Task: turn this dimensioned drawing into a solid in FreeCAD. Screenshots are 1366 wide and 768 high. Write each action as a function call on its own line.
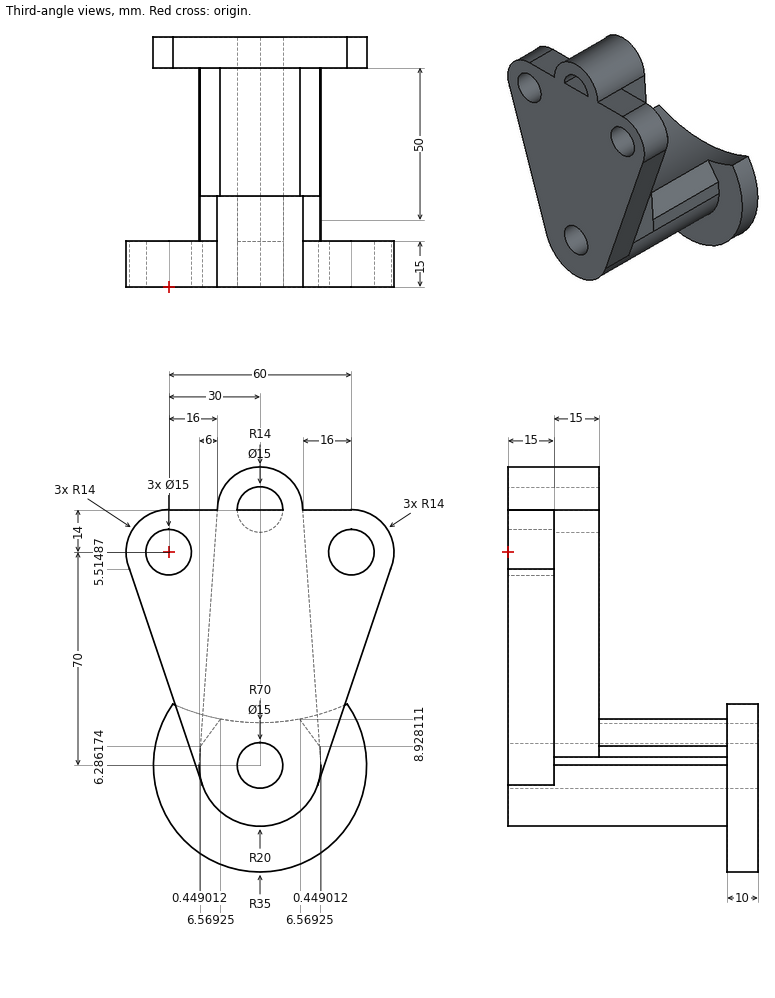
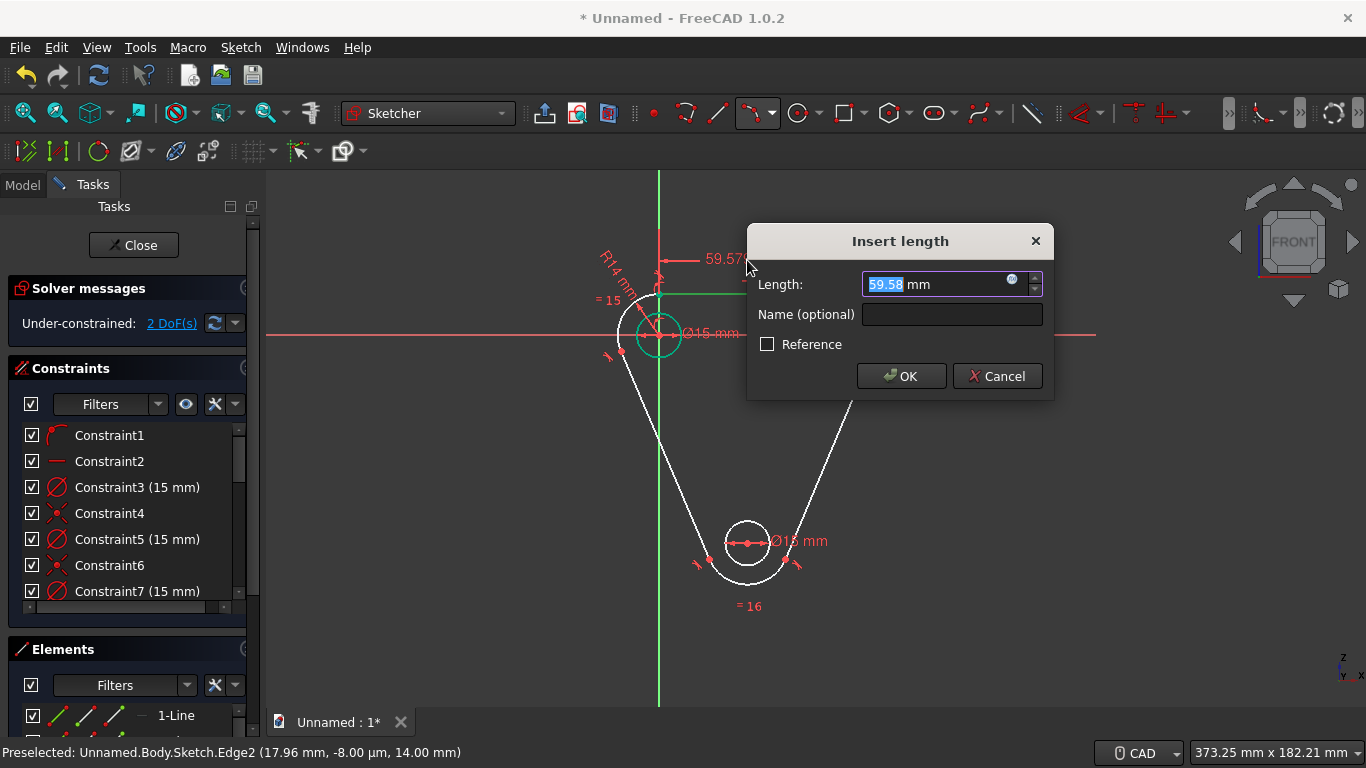
text(60)
key(Return)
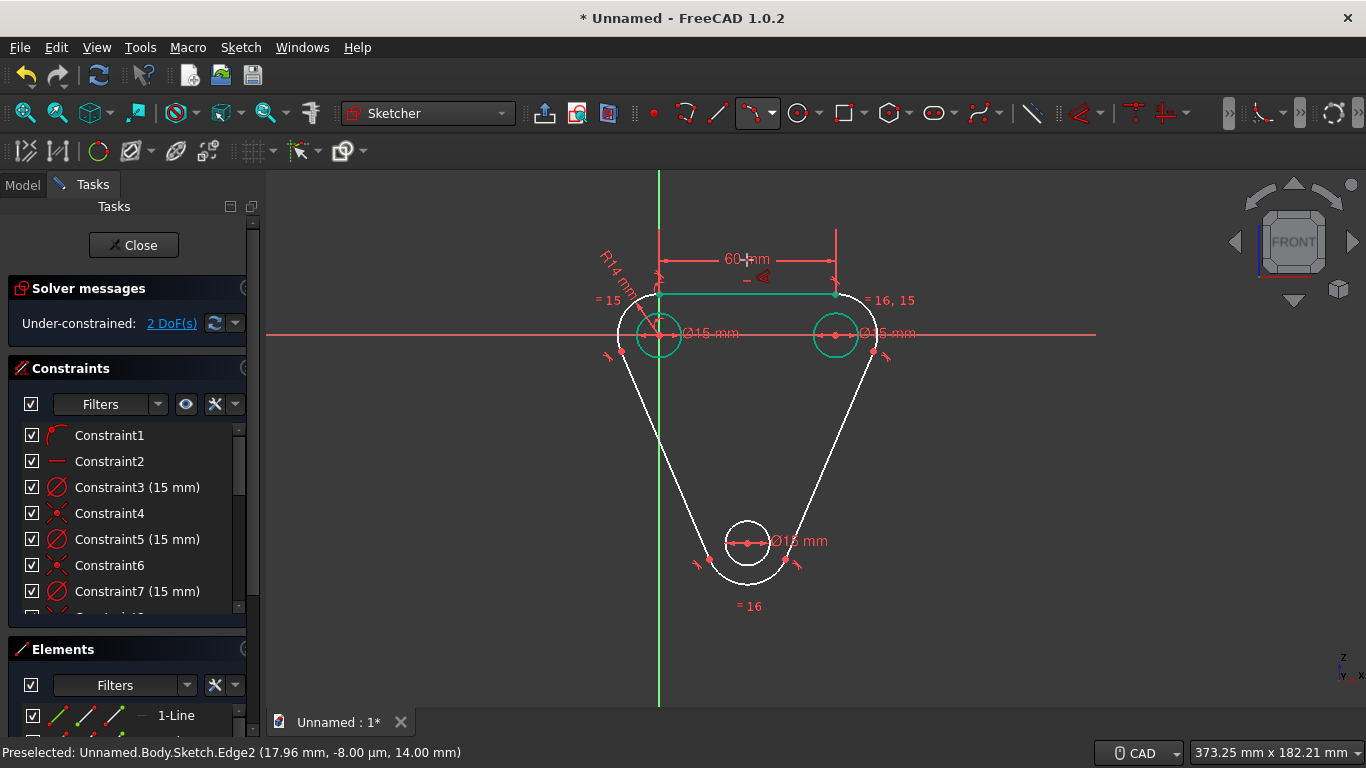
click(748, 543)
click(703, 577)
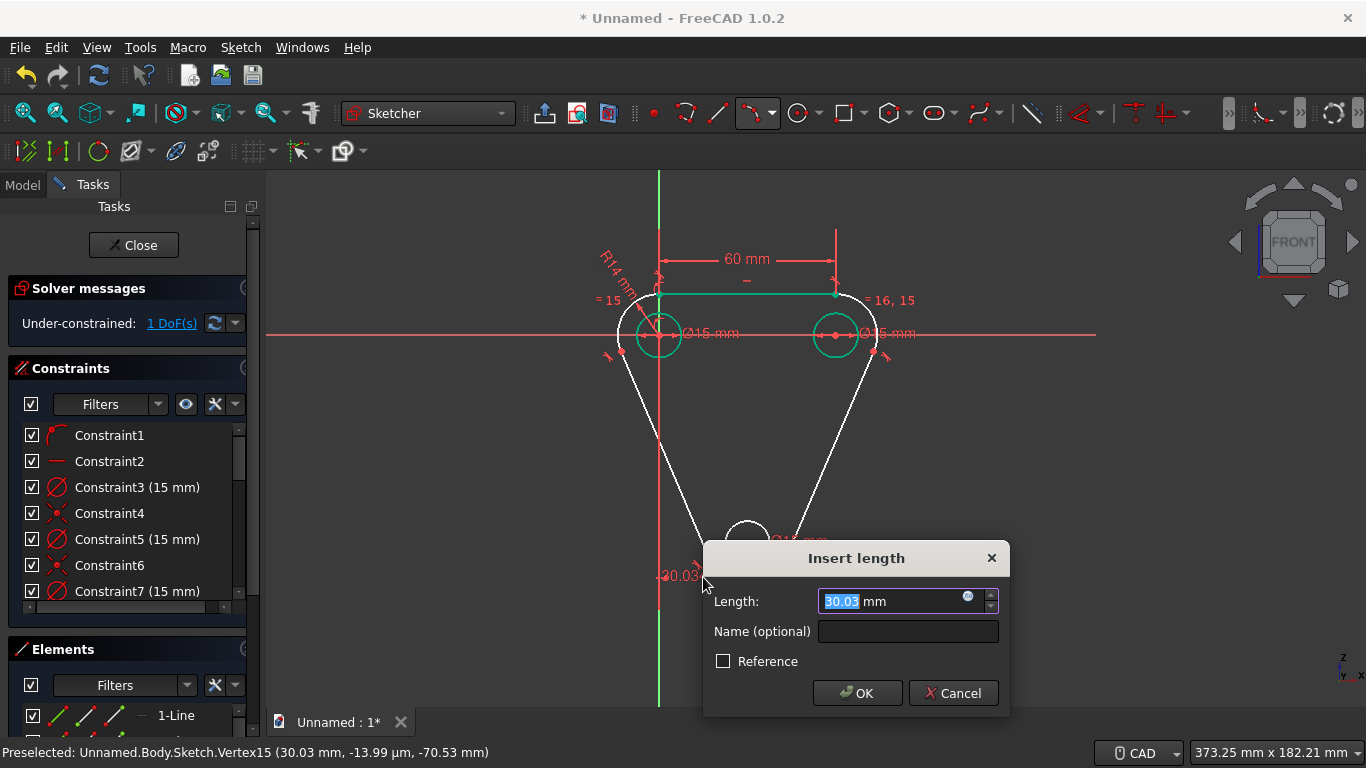
text(30)
key(Return)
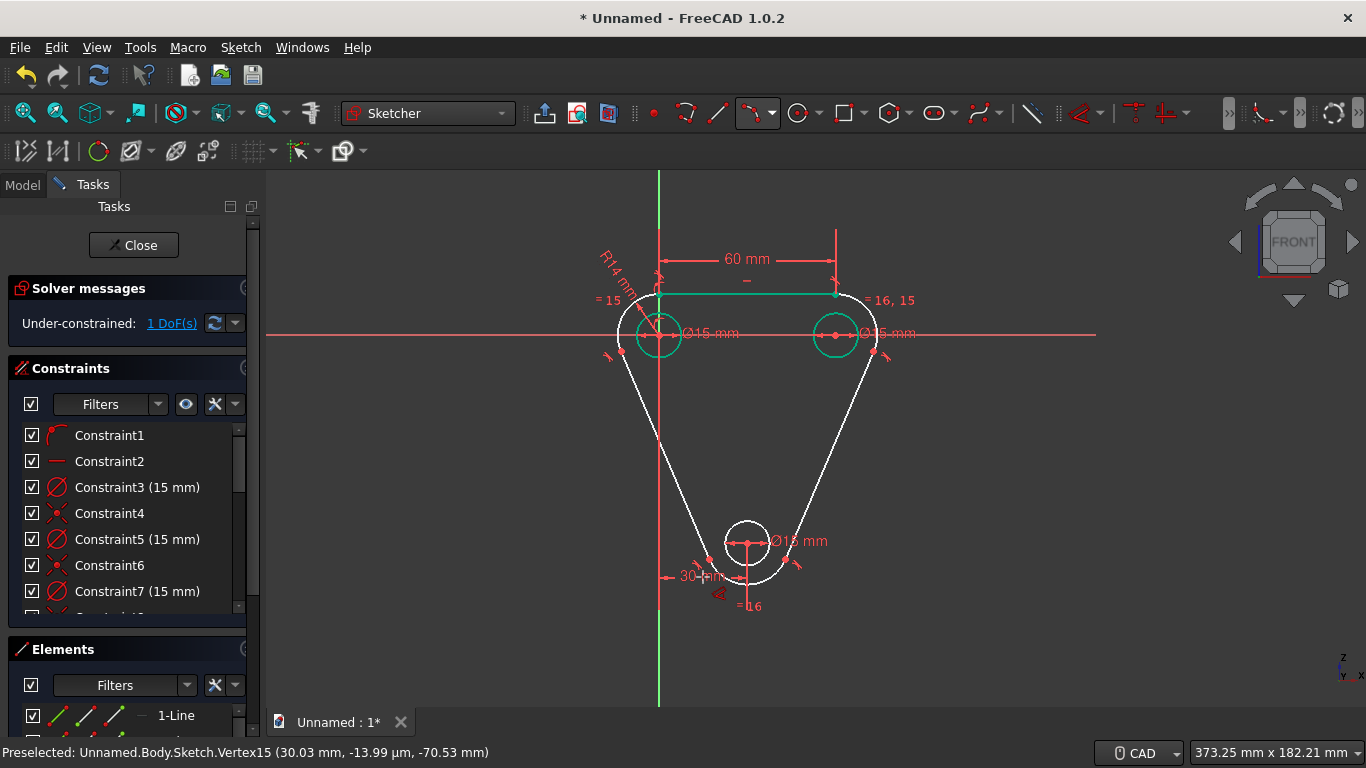
click(747, 543)
click(625, 439)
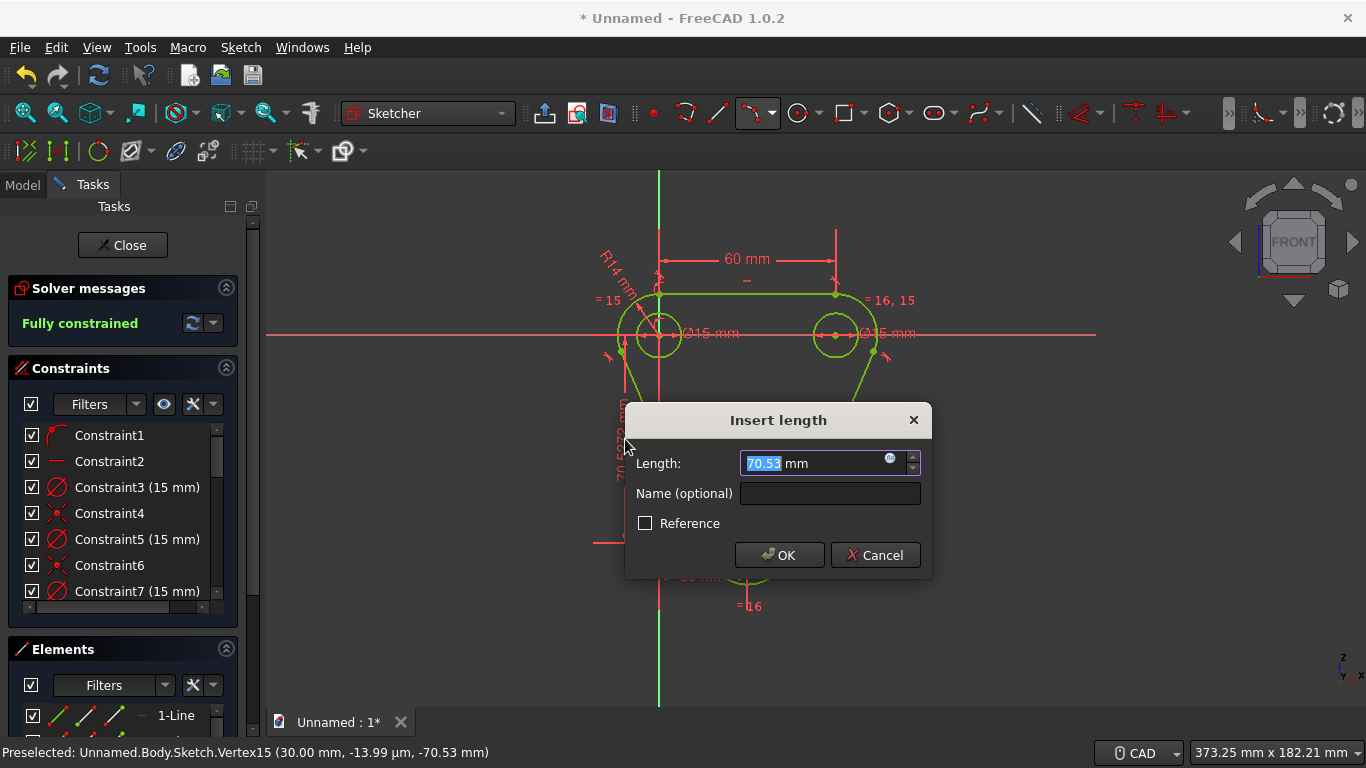
text(70)
key(Return)
key(Escape)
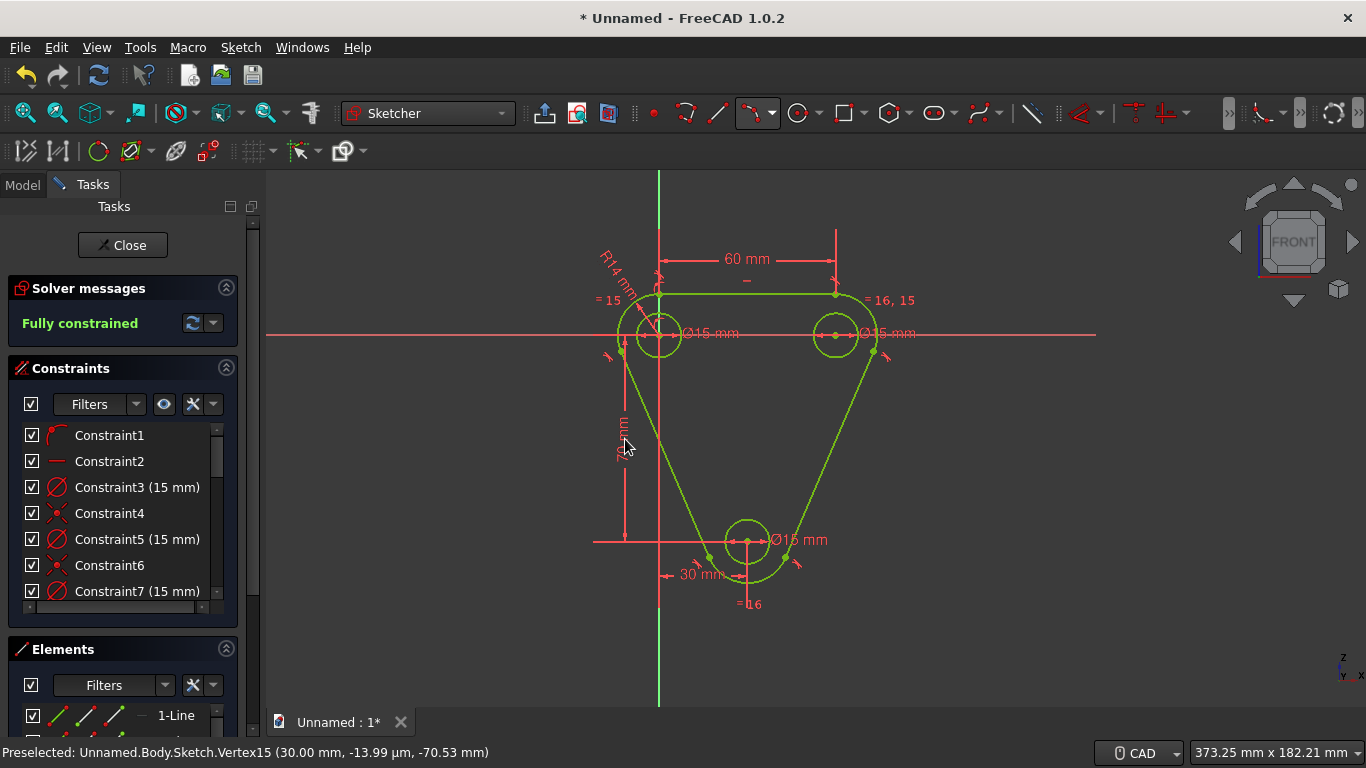
click(123, 245)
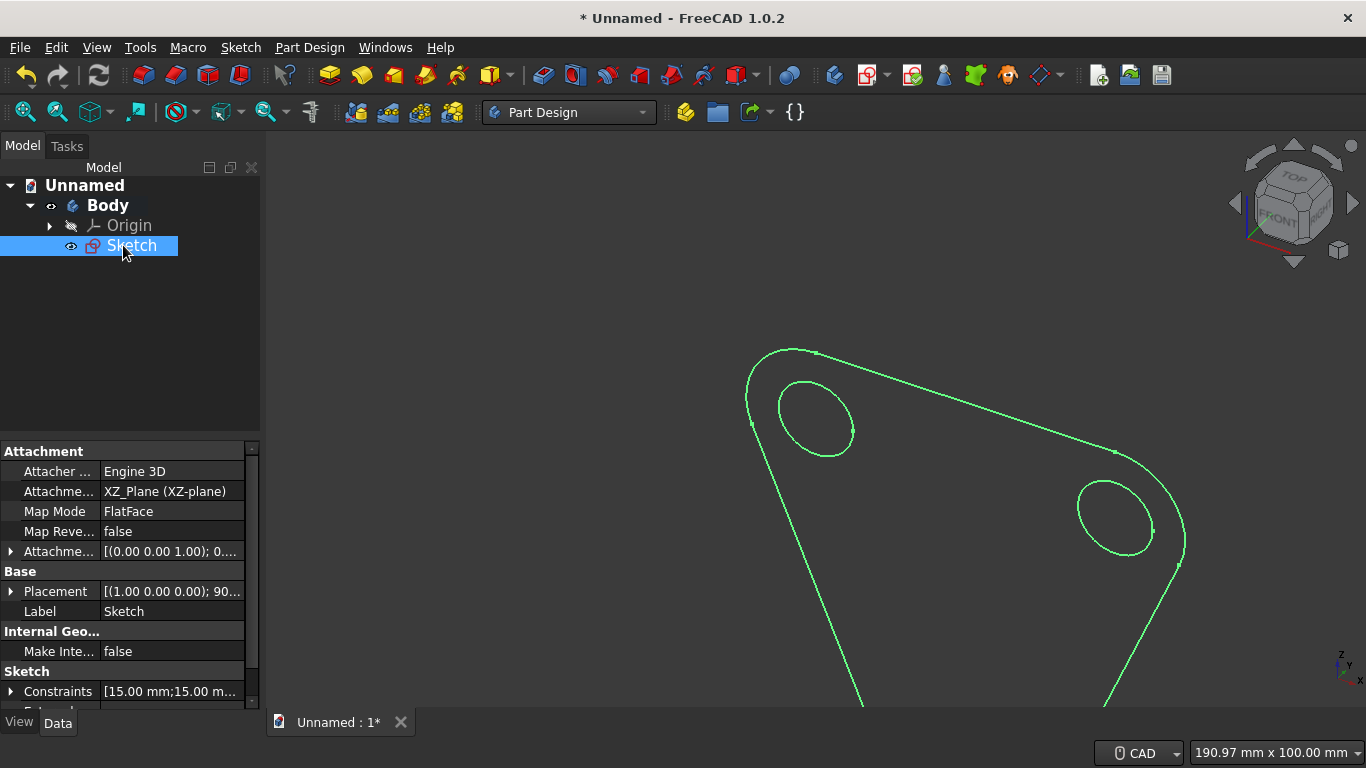
click(330, 76)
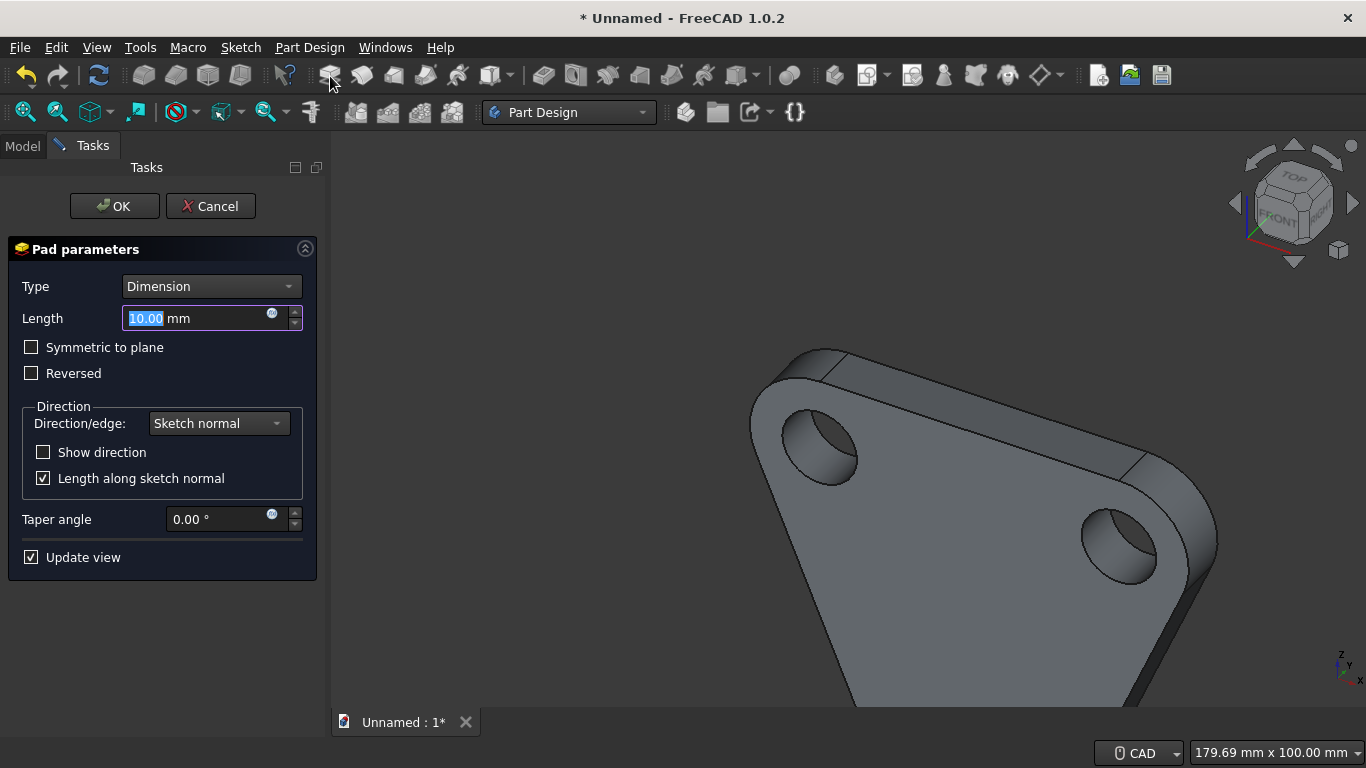
text(15)
key(Tab)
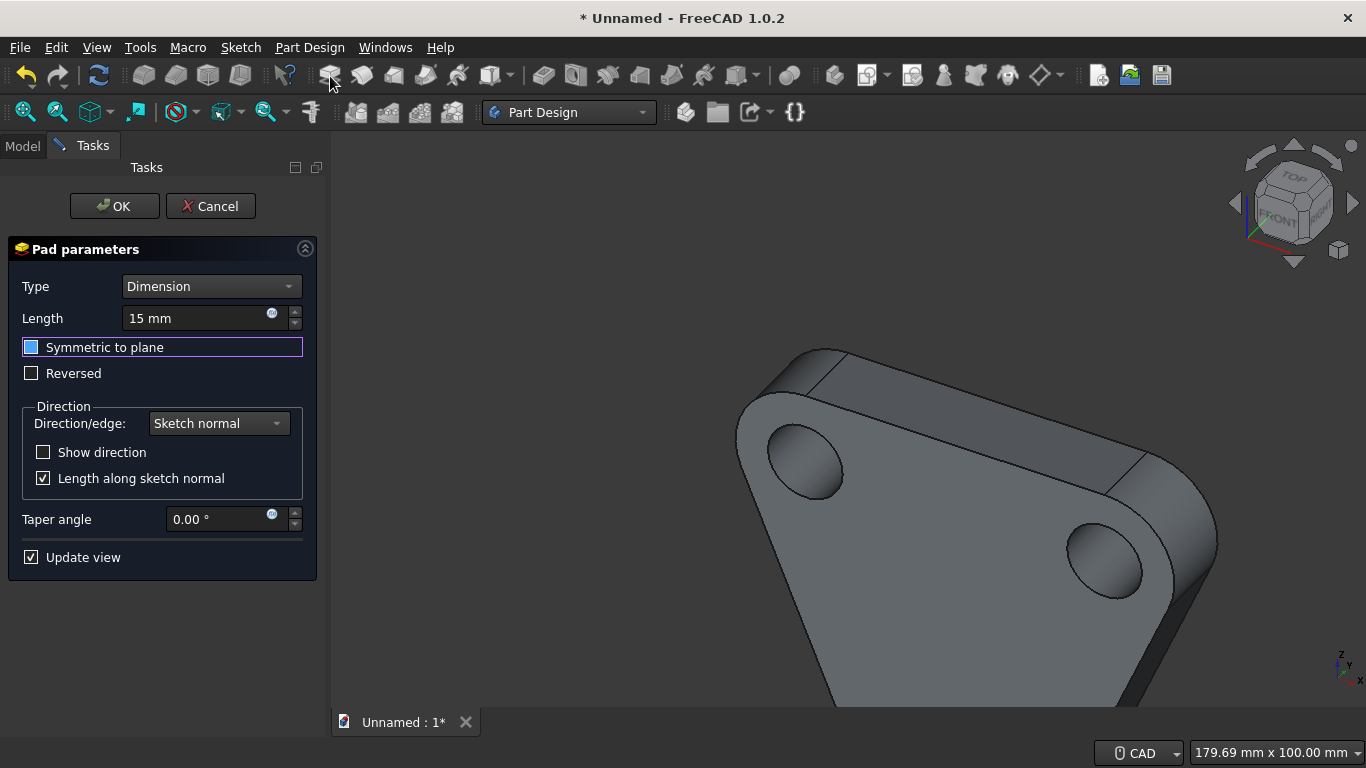
click(30, 373)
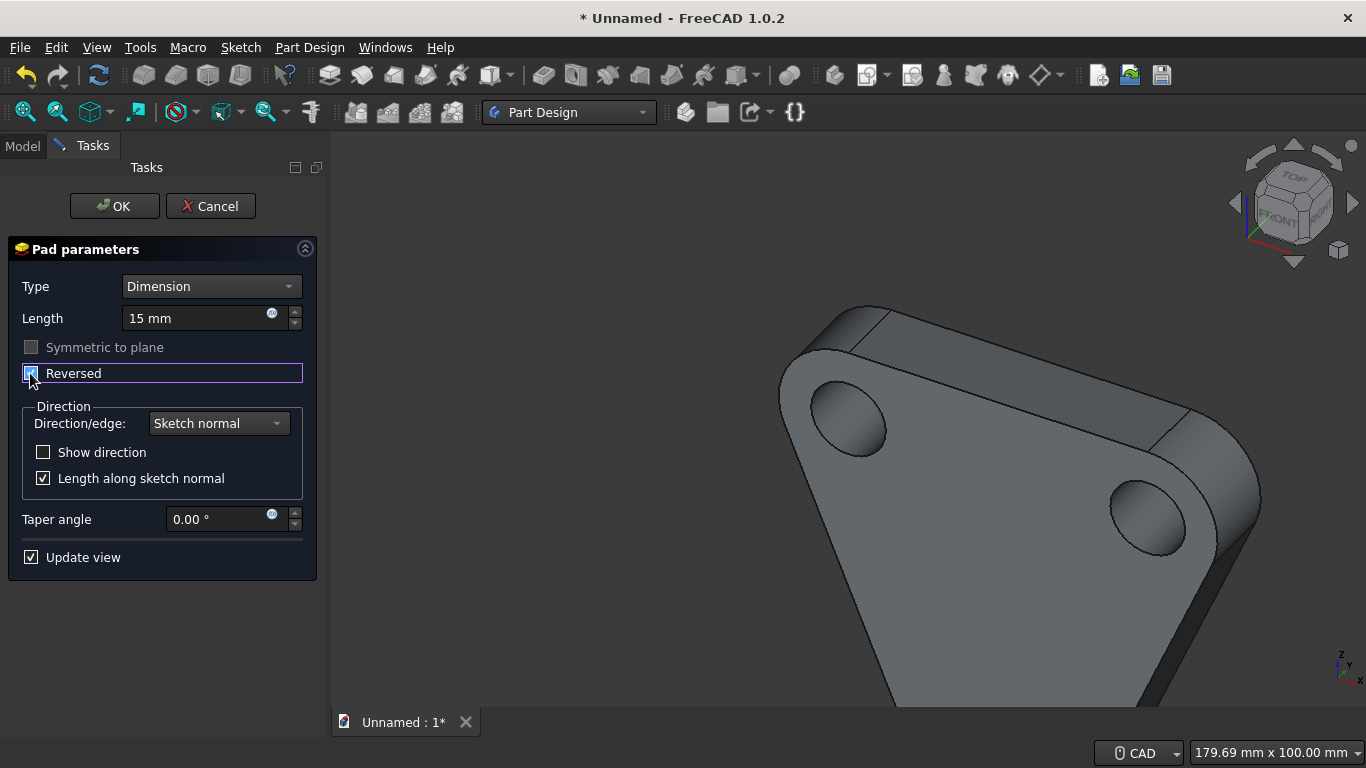
click(115, 206)